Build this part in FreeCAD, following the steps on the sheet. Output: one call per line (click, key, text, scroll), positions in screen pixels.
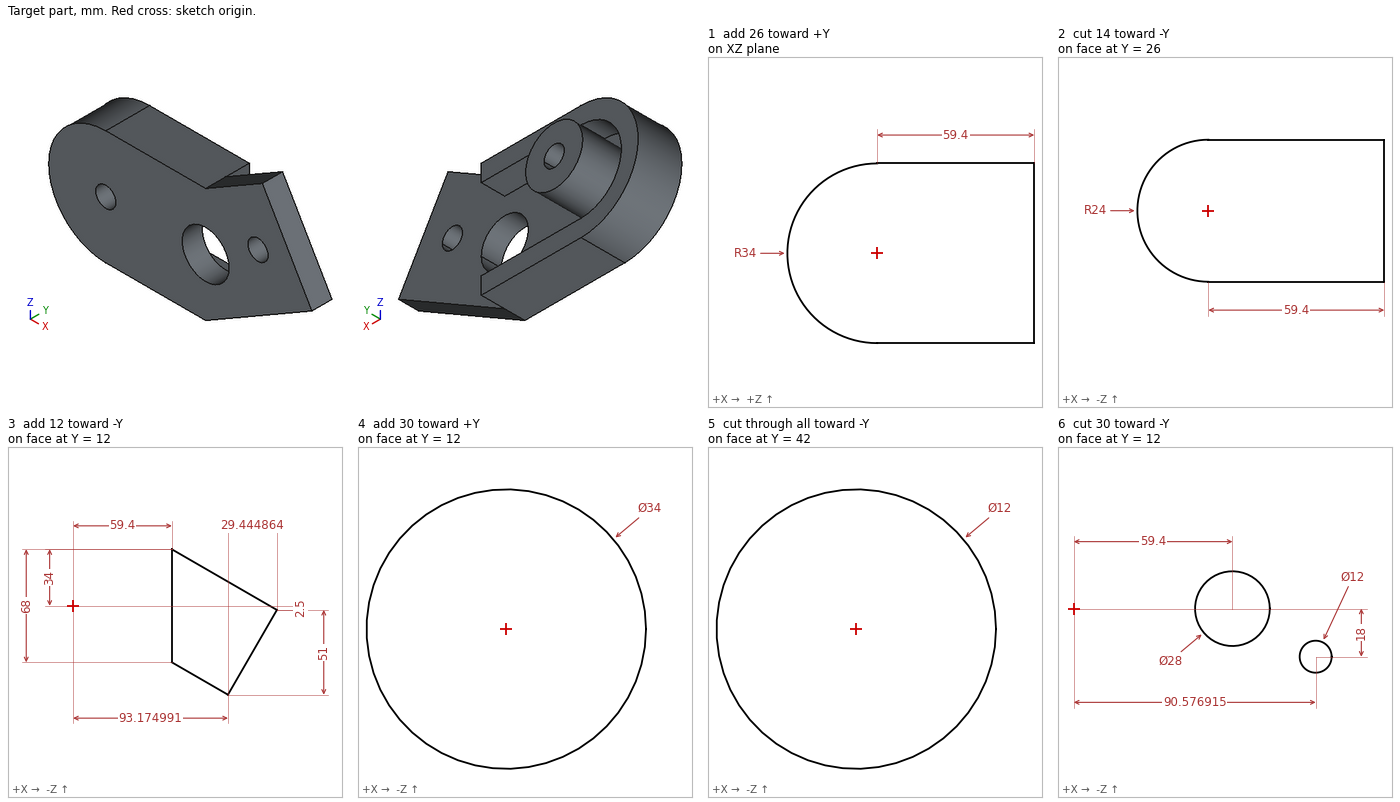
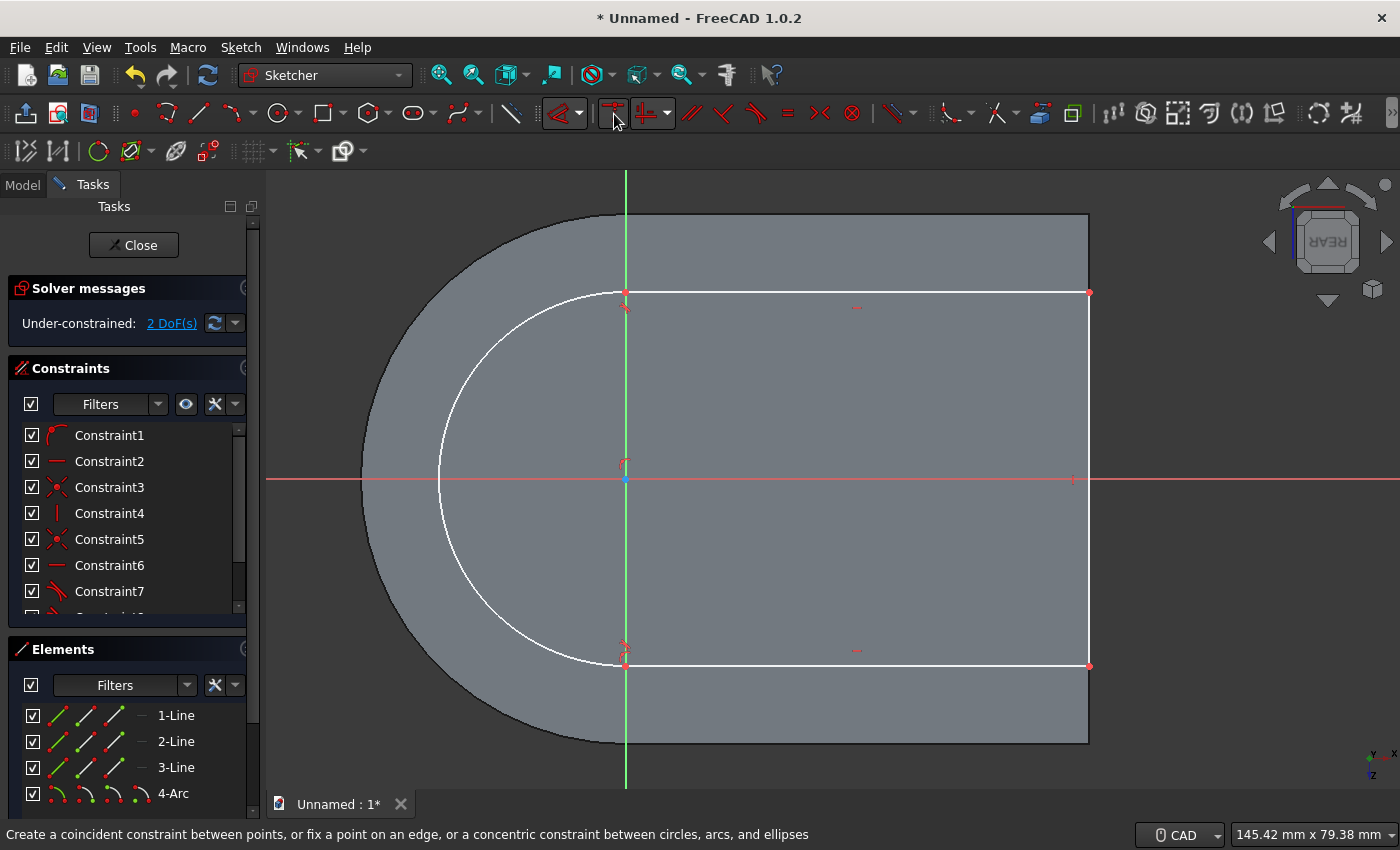
click(475, 369)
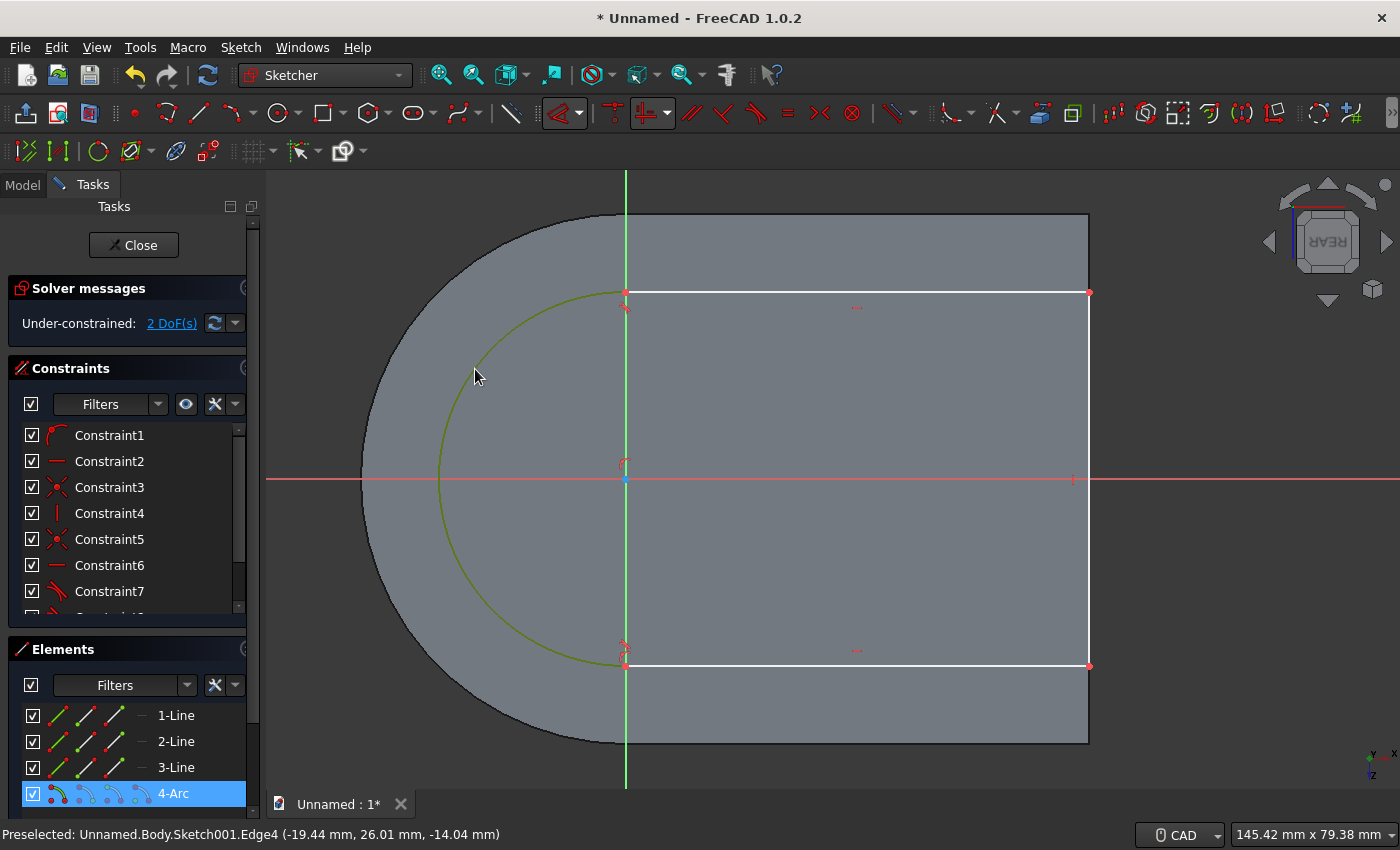
click(582, 114)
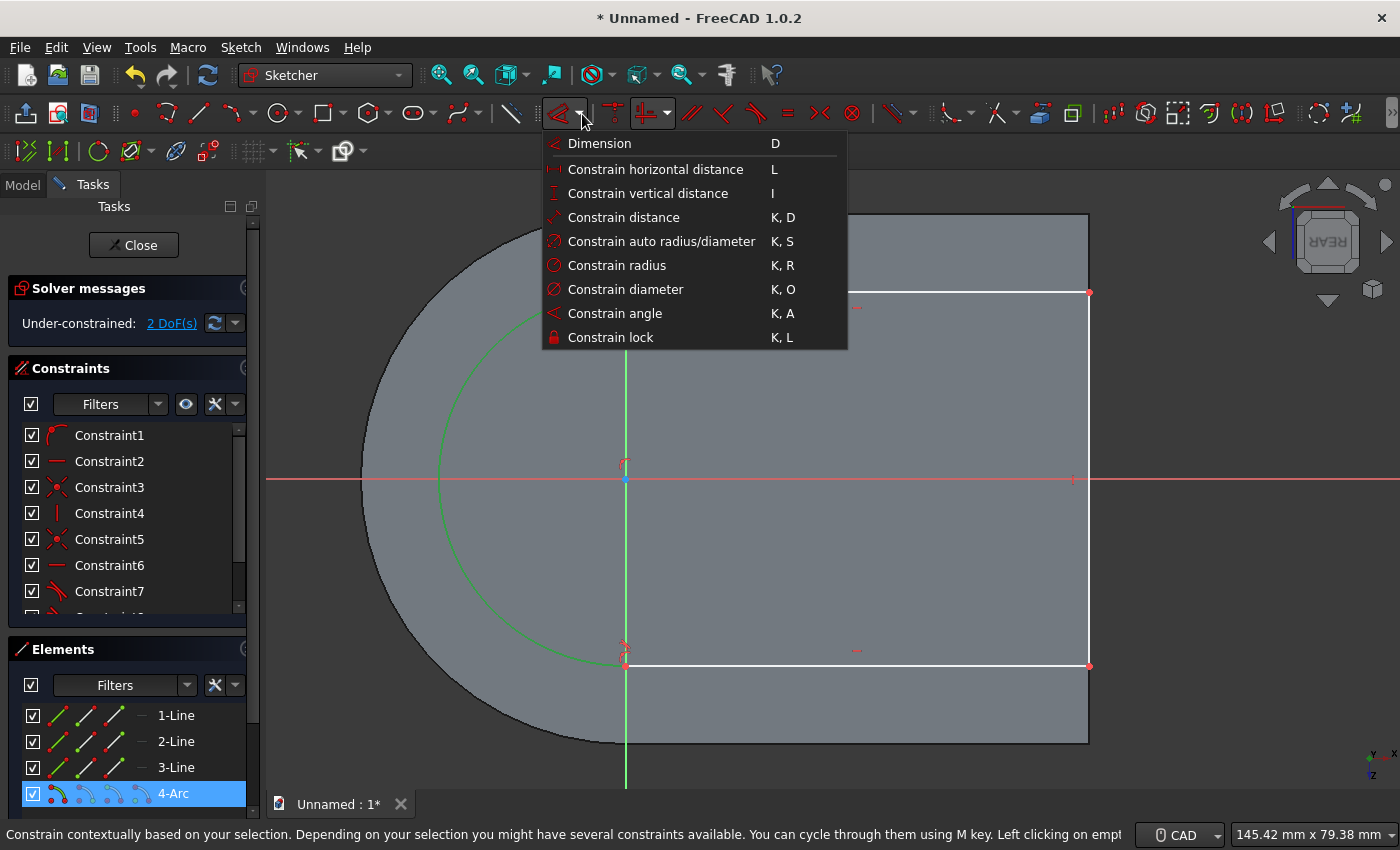
click(695, 265)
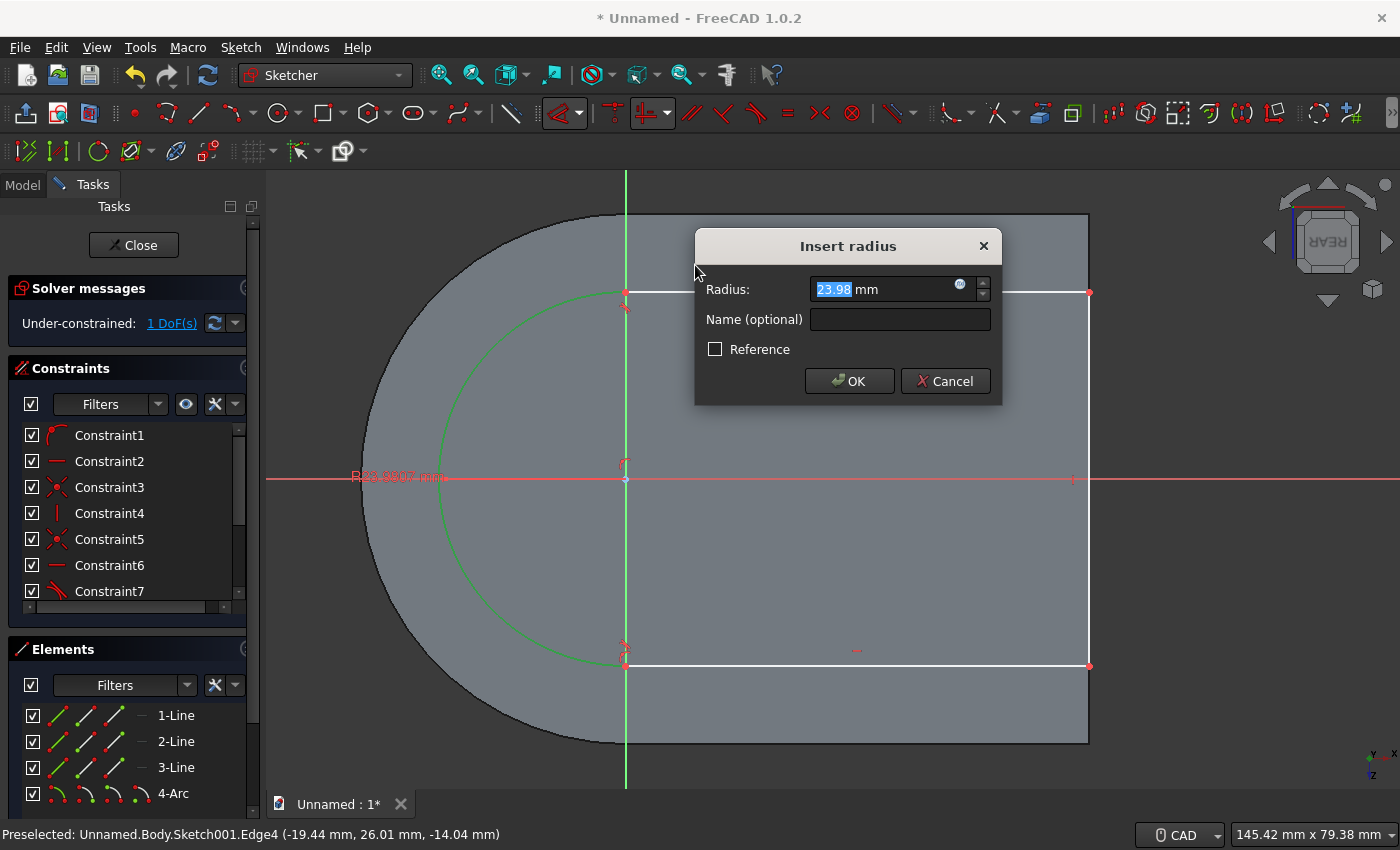
text(24)
key(Return)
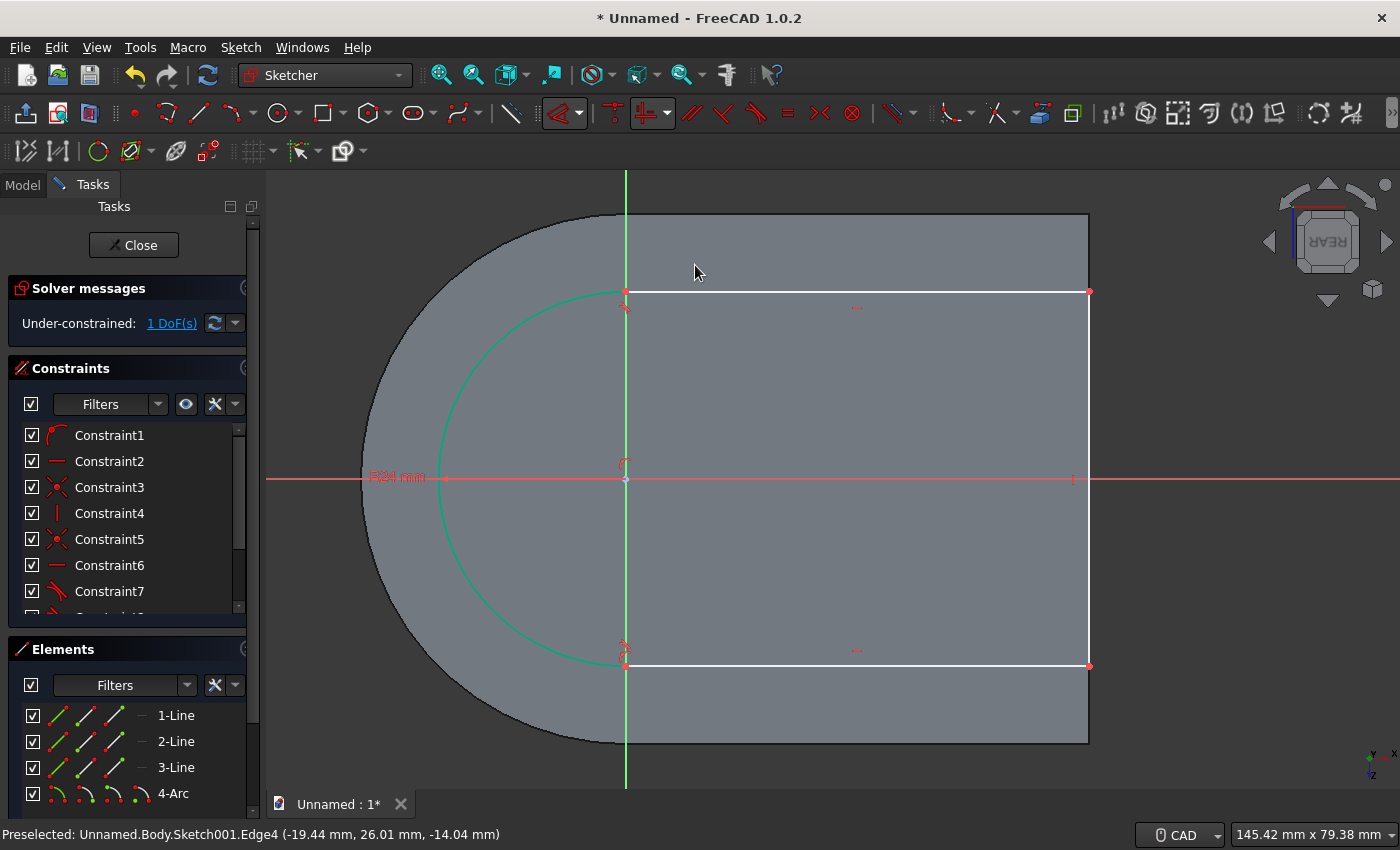
click(765, 666)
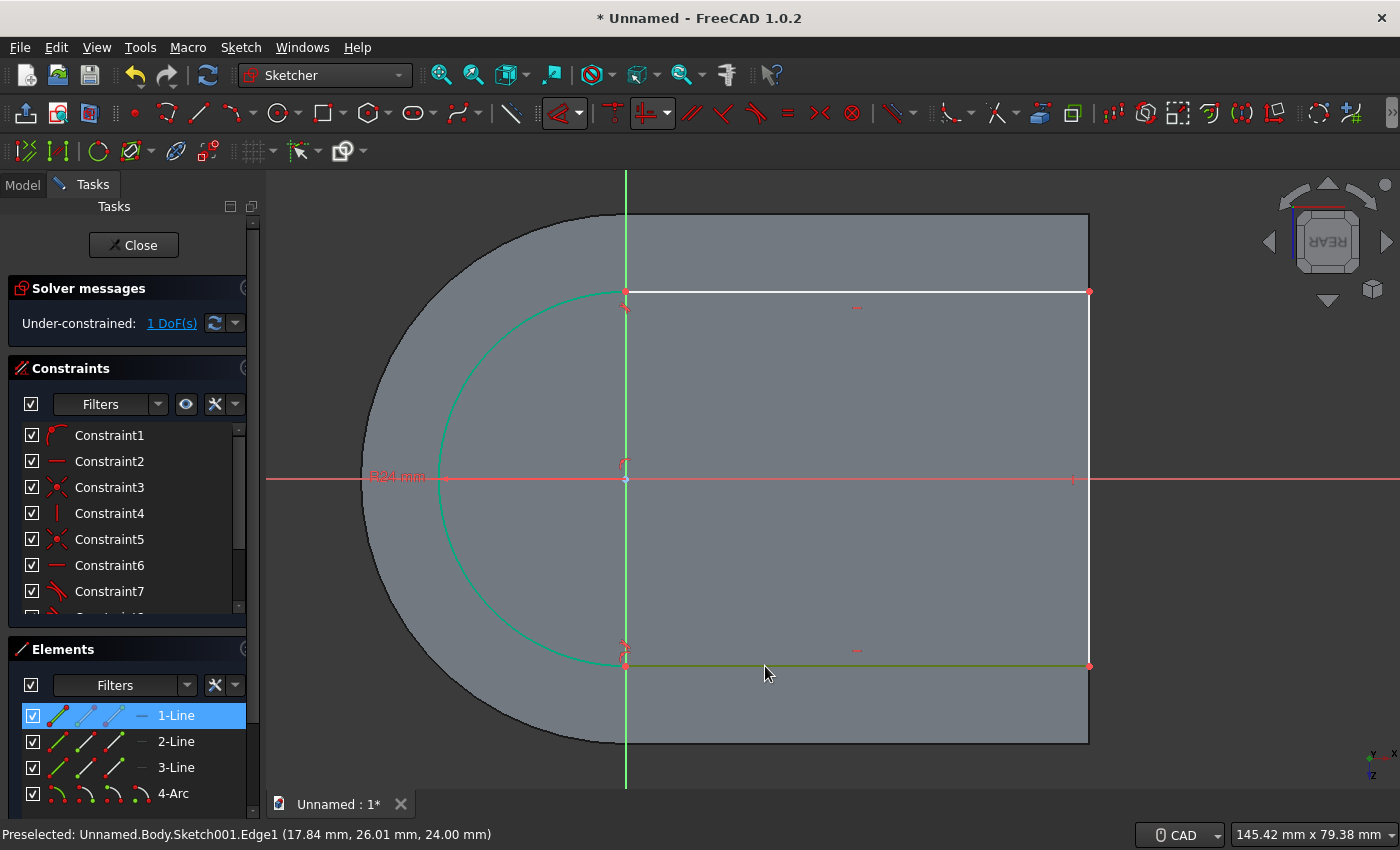
key(l)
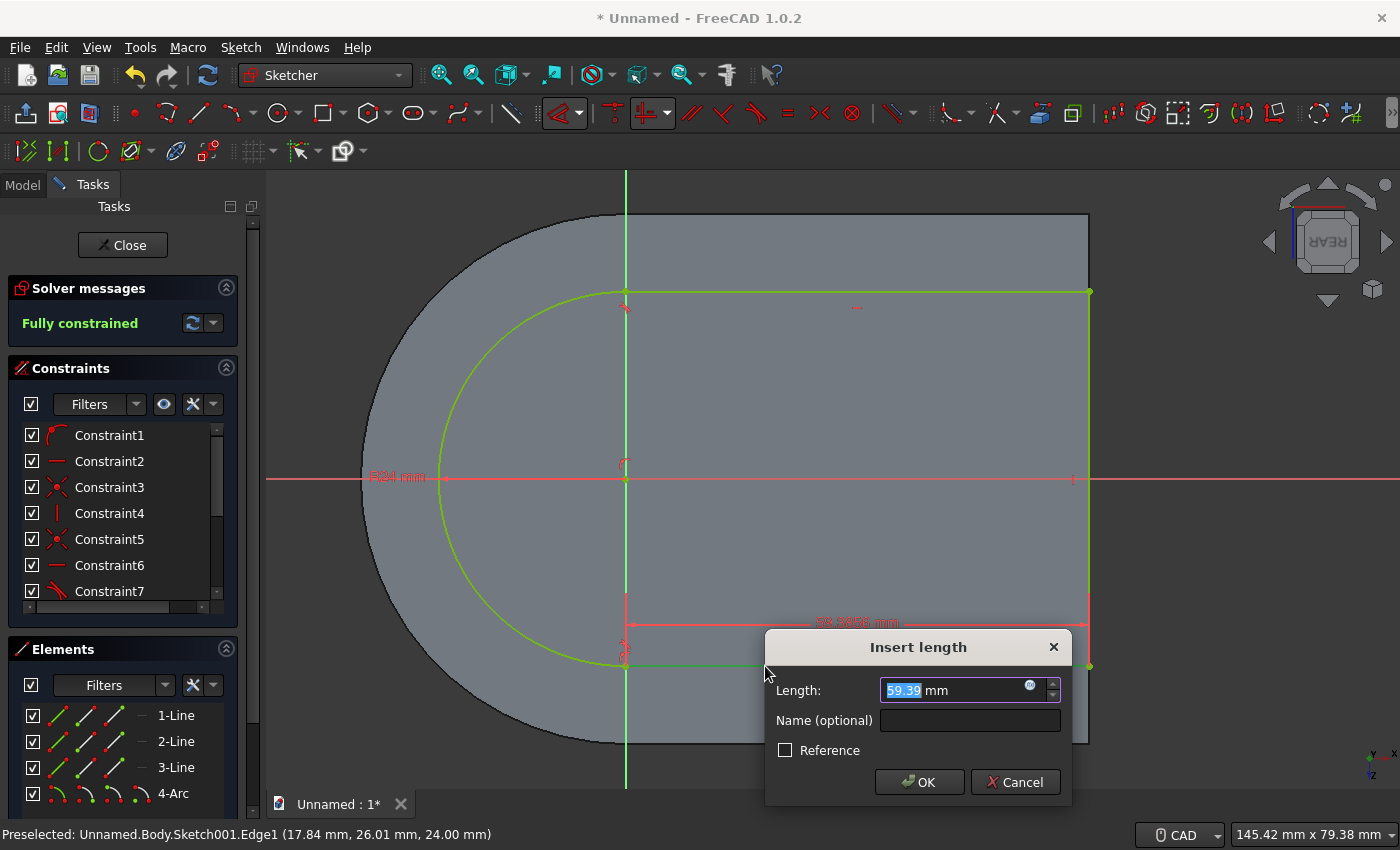
text(59.4)
key(Return)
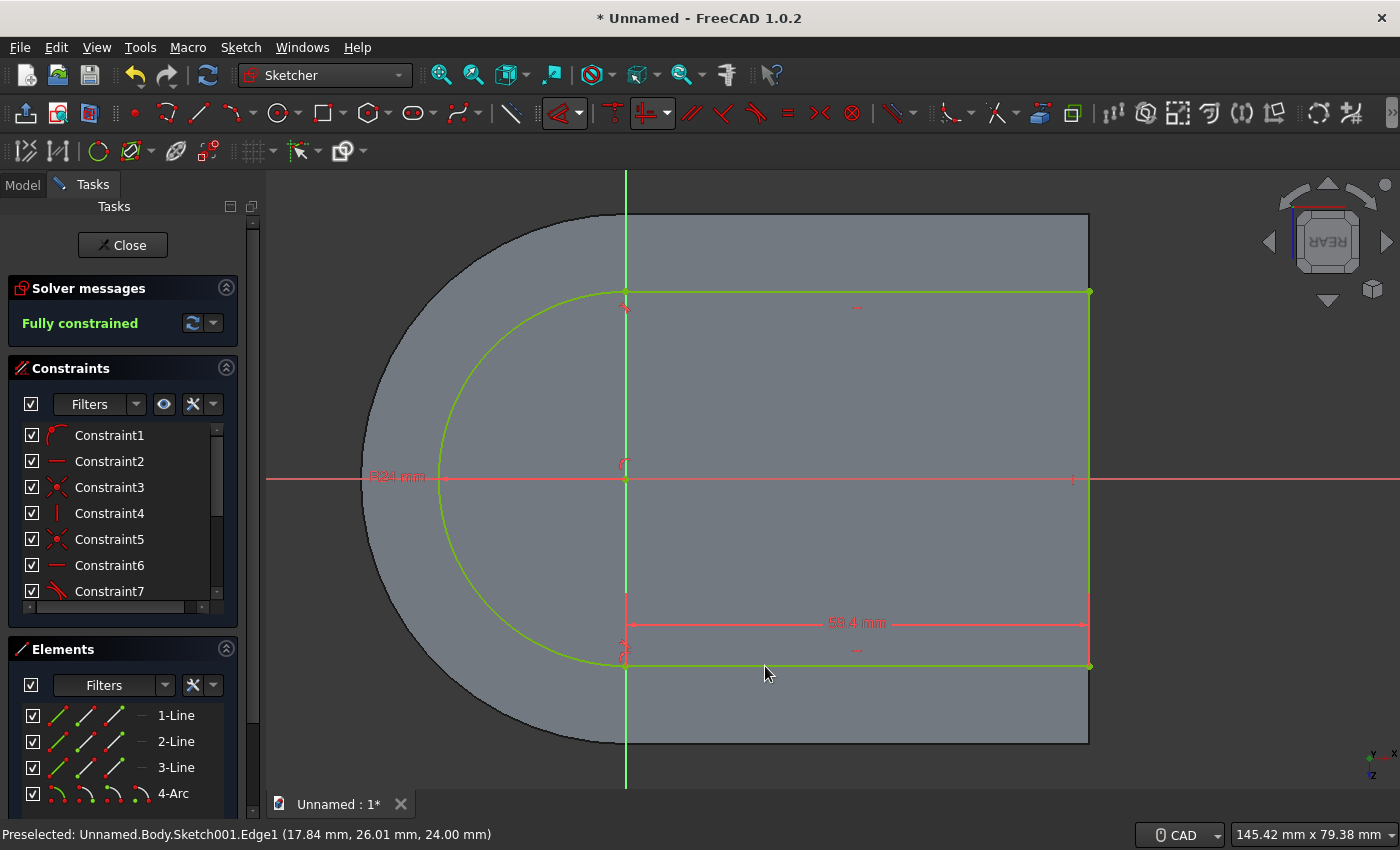
click(123, 245)